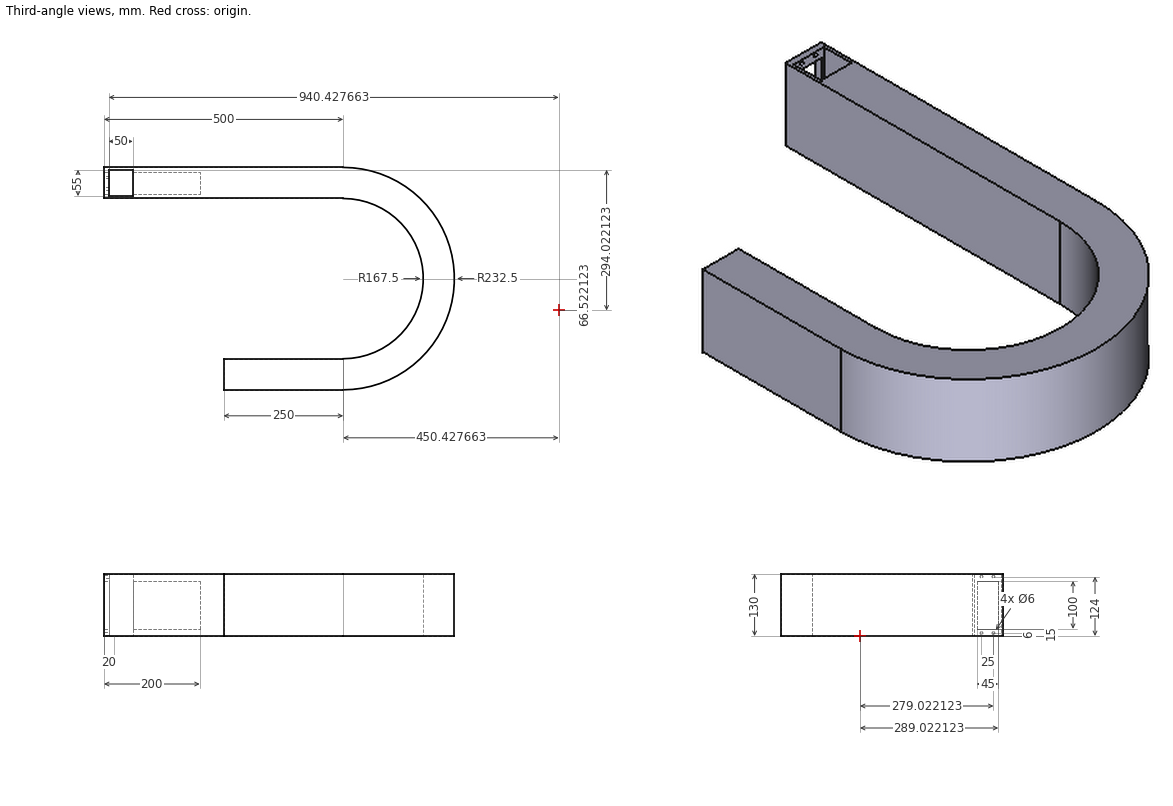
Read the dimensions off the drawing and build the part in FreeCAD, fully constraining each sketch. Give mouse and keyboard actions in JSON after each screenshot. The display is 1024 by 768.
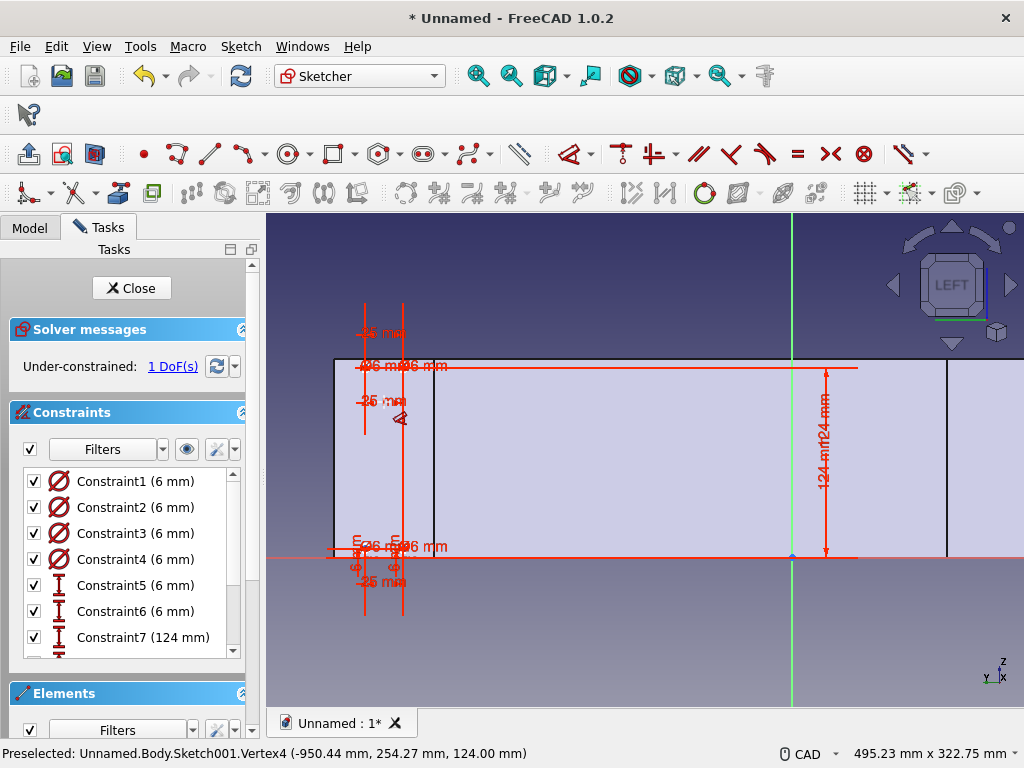
{"action": "left_click", "coordinate": [365, 549]}
{"action": "left_click", "coordinate": [579, 592]}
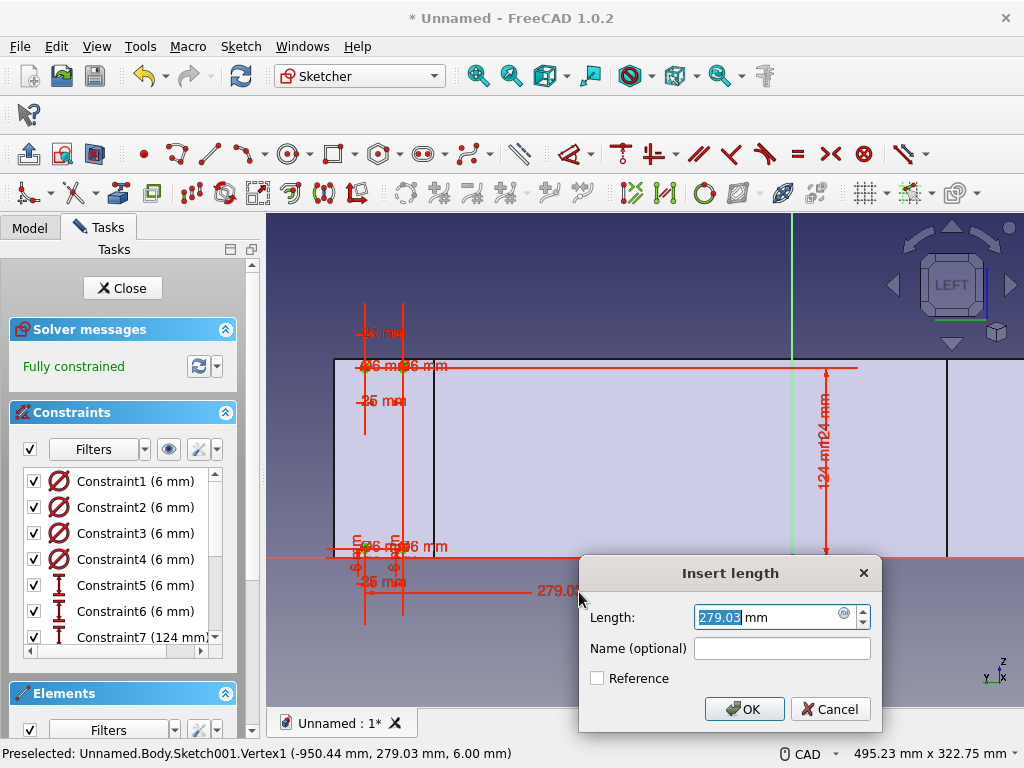
{"action": "type", "text": "279.022123"}
{"action": "key", "text": "Return"}
{"action": "key", "text": "Escape"}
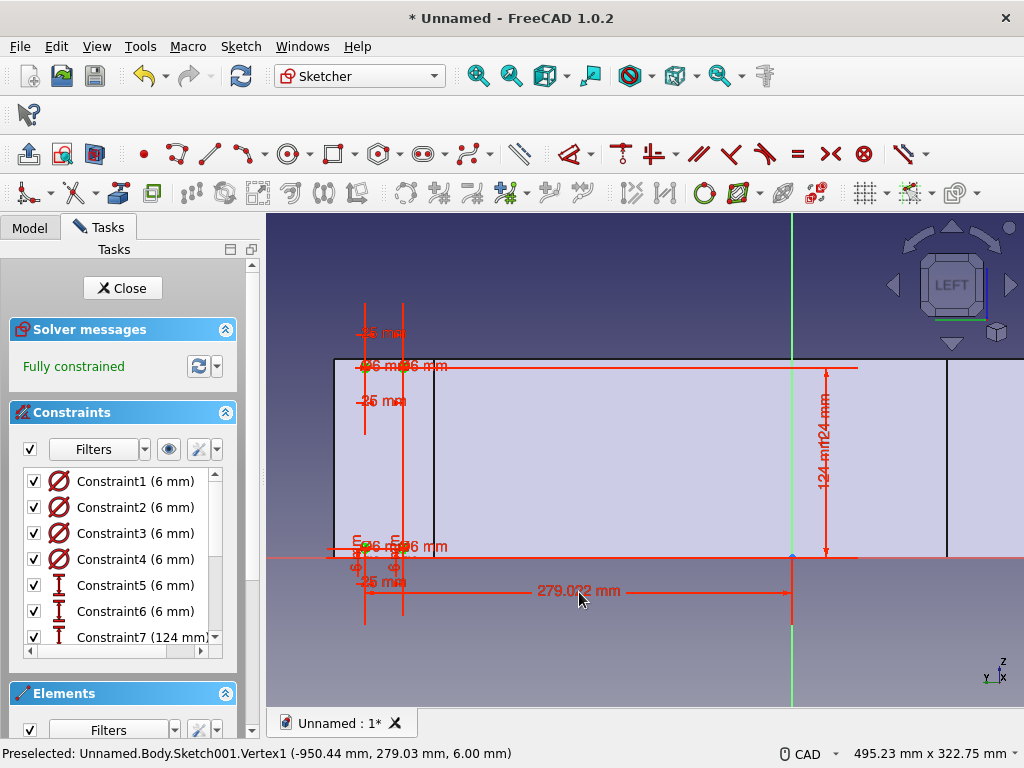
{"action": "left_click", "coordinate": [123, 288]}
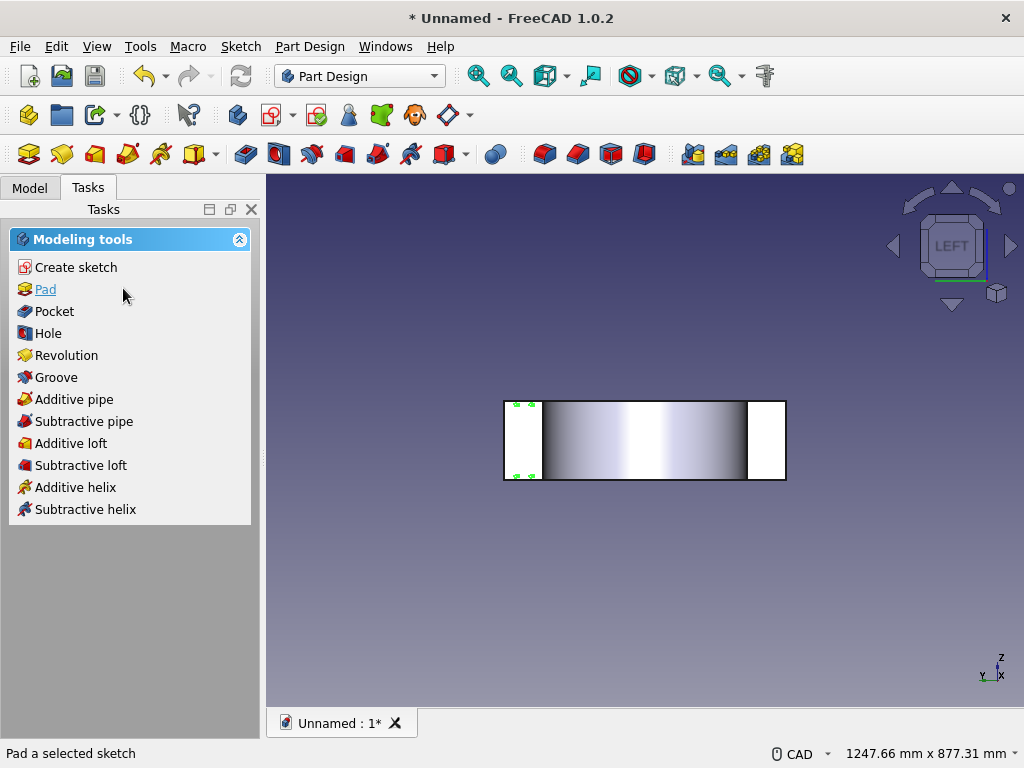
{"action": "left_click", "coordinate": [246, 154]}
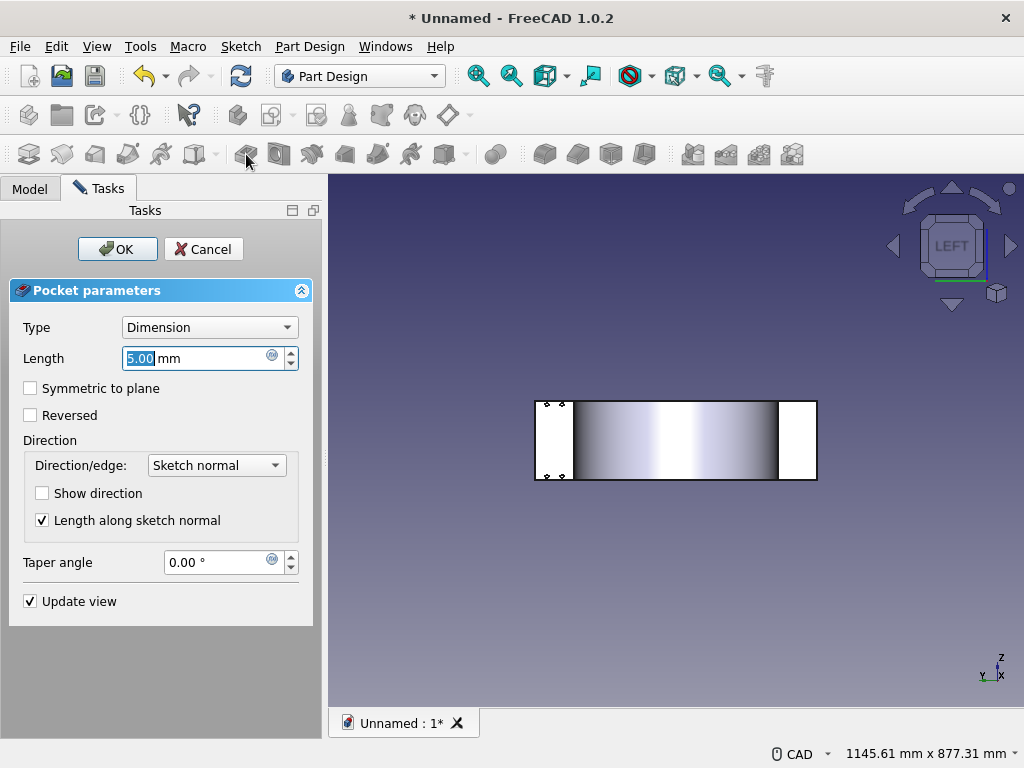
{"action": "type", "text": "20"}
{"action": "key", "text": "Tab"}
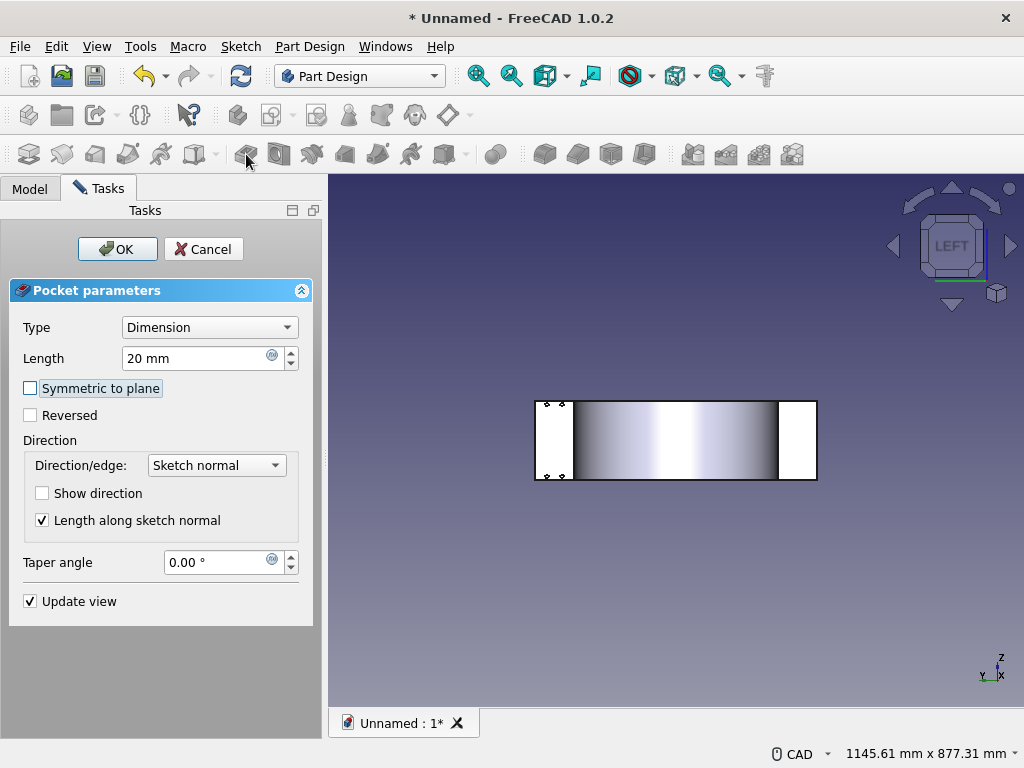
{"action": "left_click", "coordinate": [118, 249]}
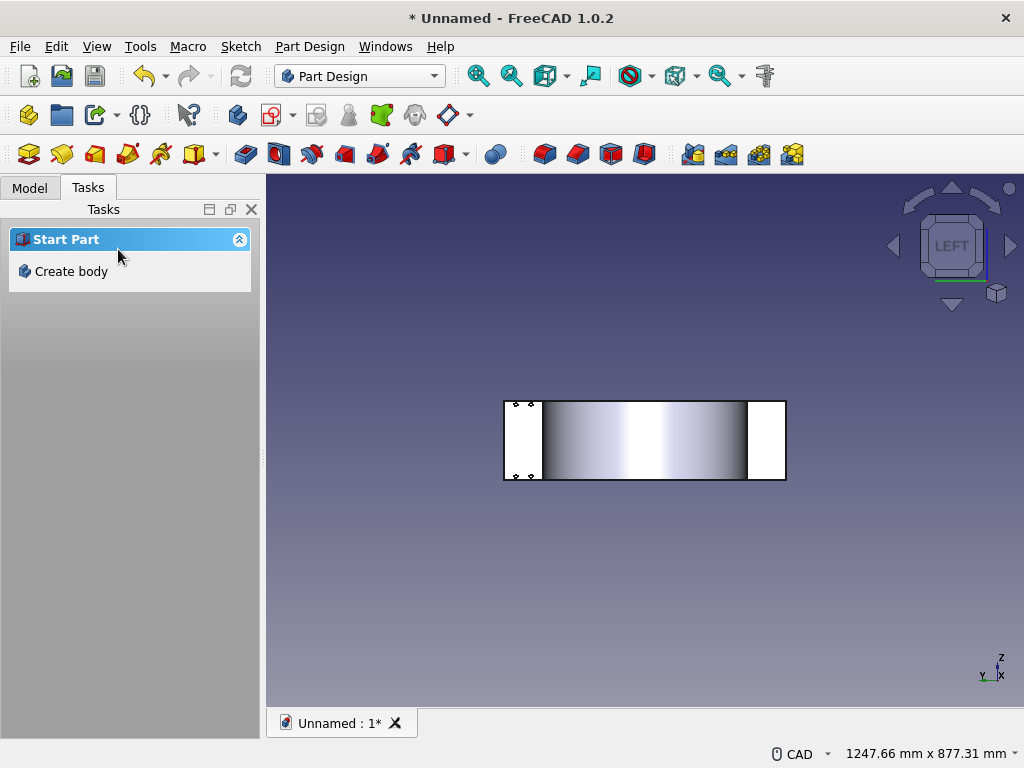
{"action": "key", "text": "v f"}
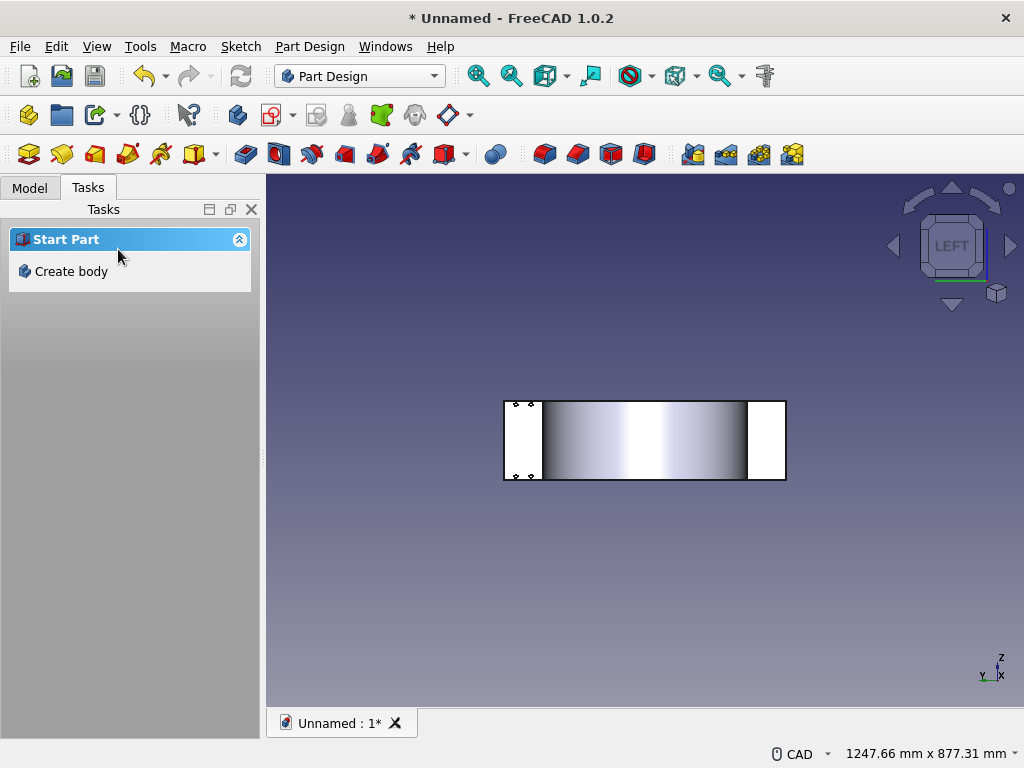
{"action": "key", "text": "0"}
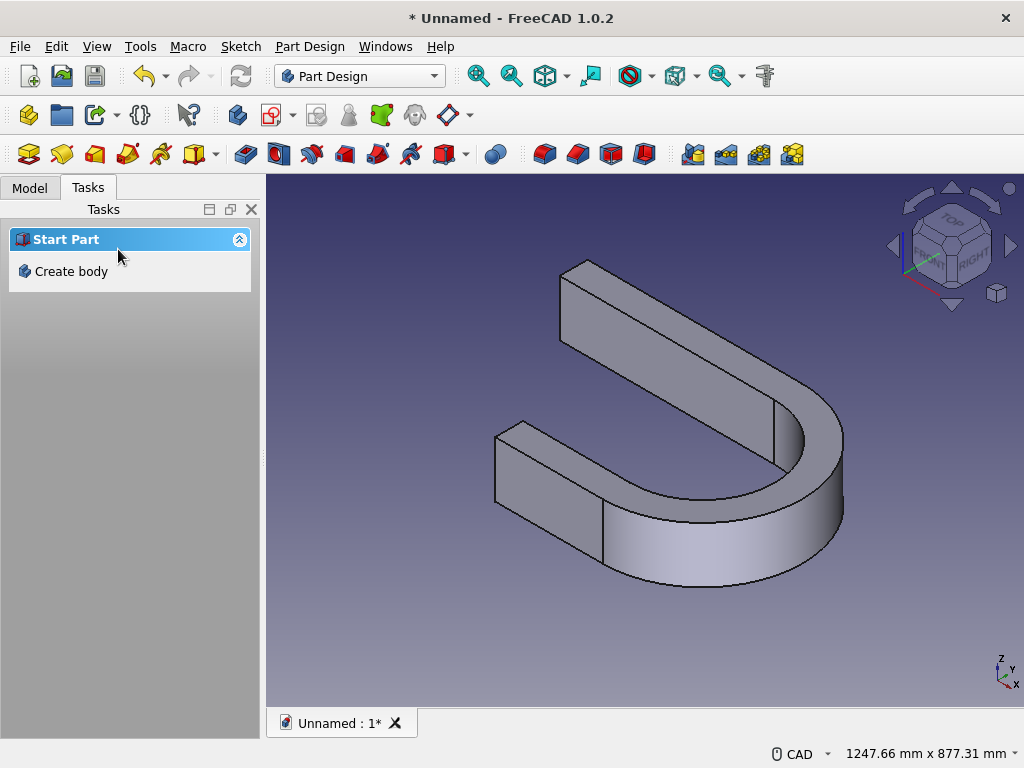
{"action": "left_click", "coordinate": [776, 384]}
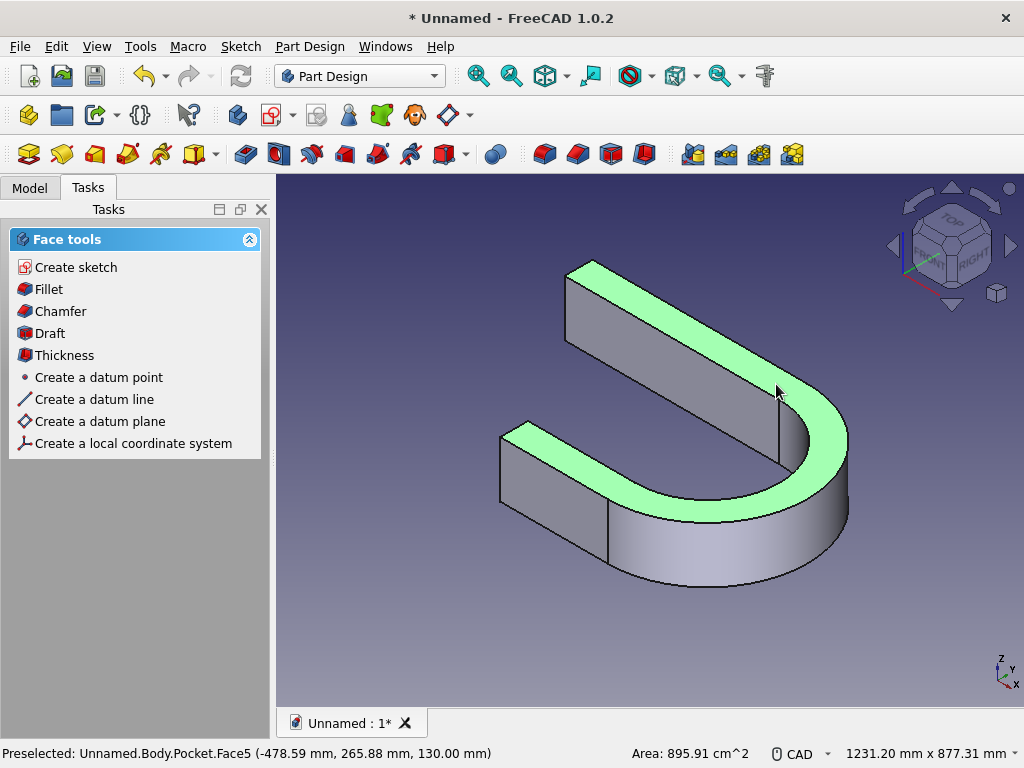
{"action": "left_click", "coordinate": [270, 116]}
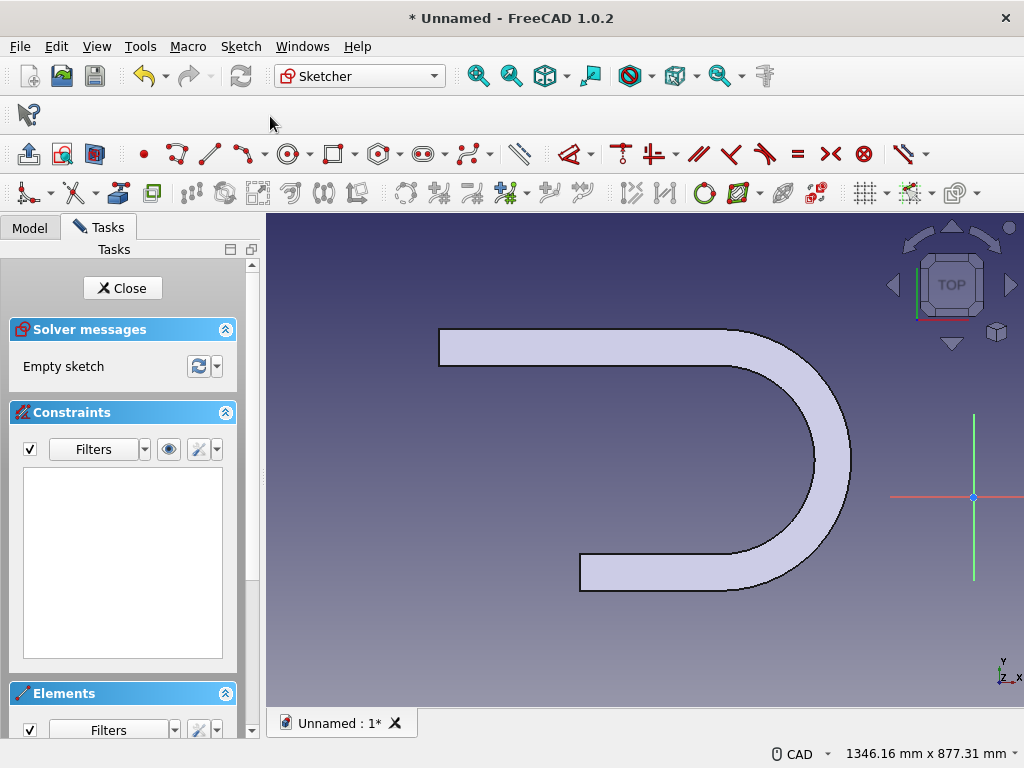
{"action": "scroll", "coordinate": [447, 336], "scroll_direction": "up", "scroll_amount": 12}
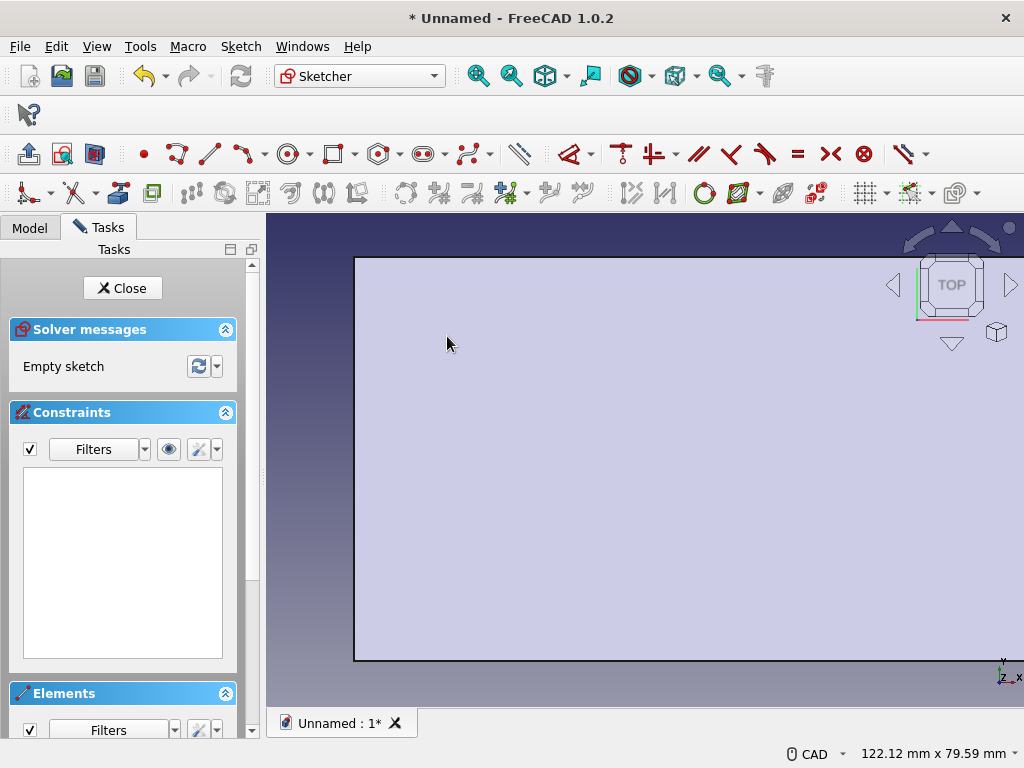
{"action": "left_click", "coordinate": [332, 154]}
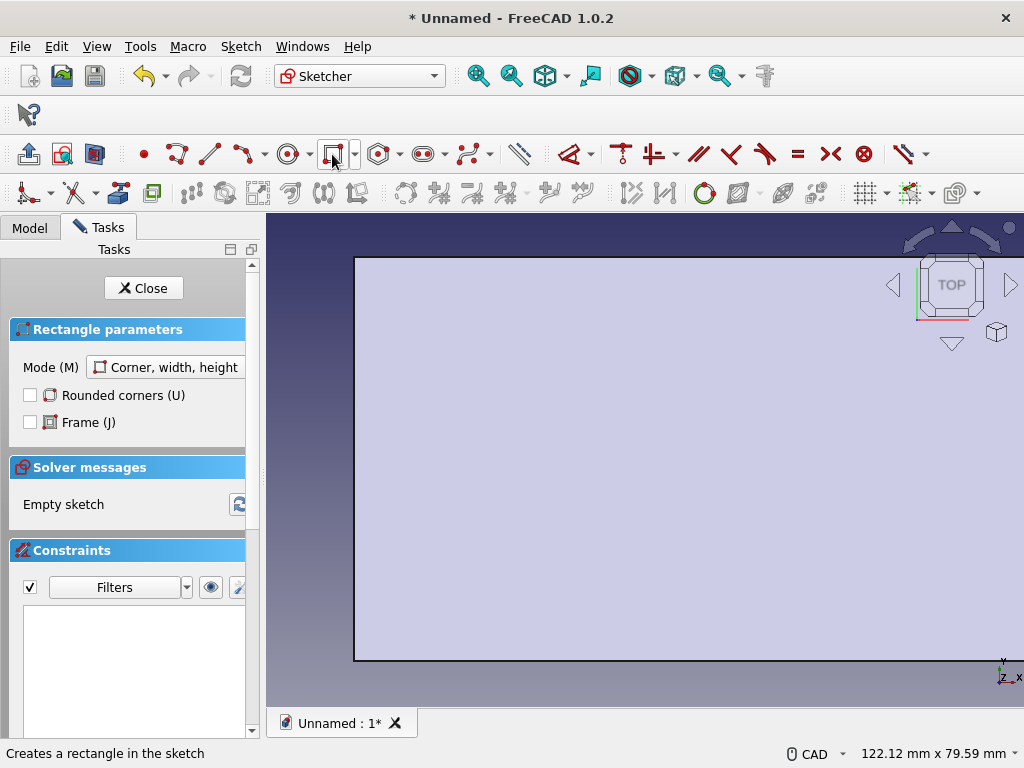
{"action": "left_click", "coordinate": [416, 288]}
{"action": "mouse_move", "coordinate": [726, 630]}